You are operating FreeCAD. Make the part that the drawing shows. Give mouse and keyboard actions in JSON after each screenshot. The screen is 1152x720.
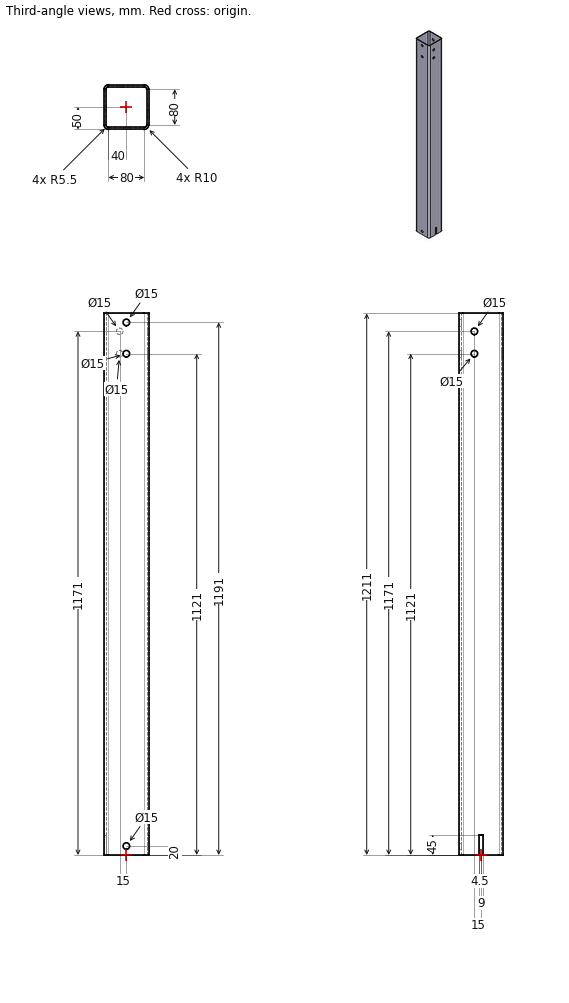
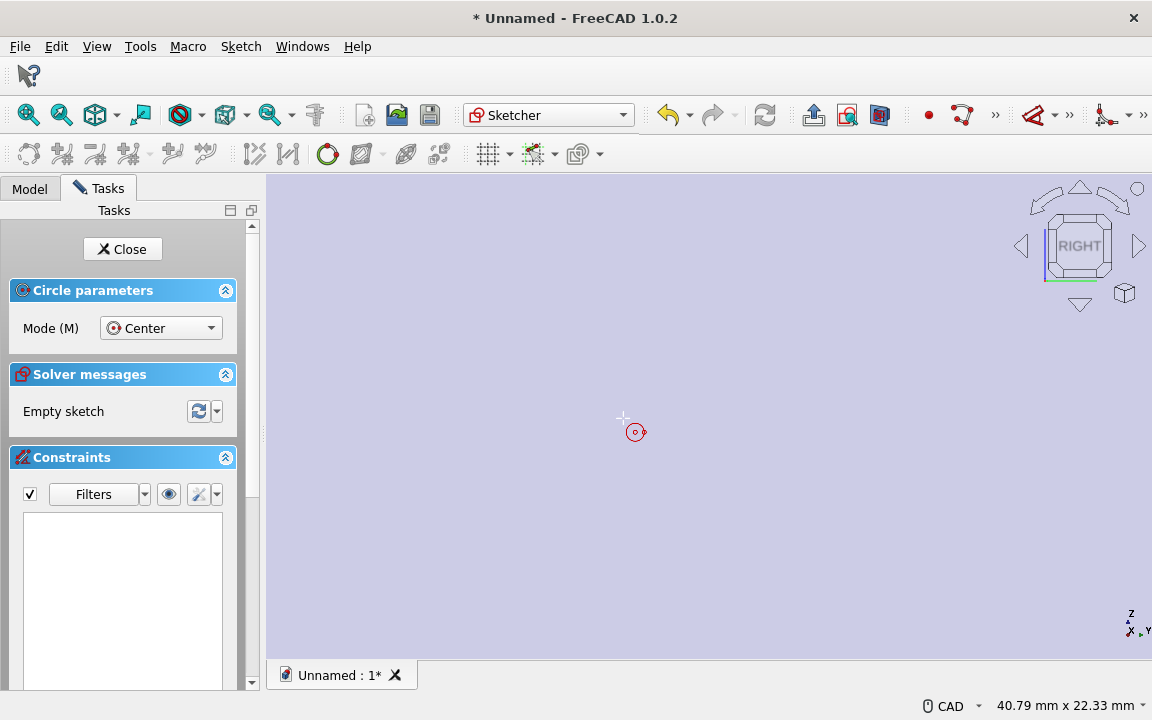
{"action": "left_click", "coordinate": [638, 416]}
{"action": "left_click", "coordinate": [753, 301]}
{"action": "key", "text": "Escape"}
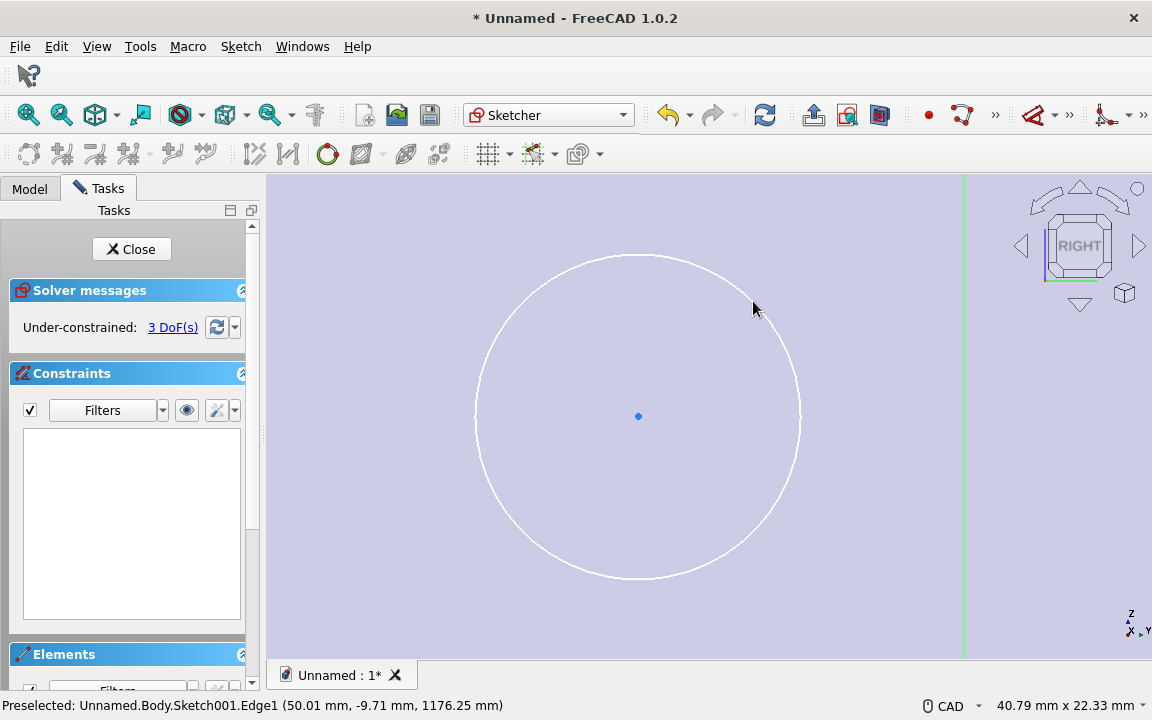
{"action": "key", "text": "d"}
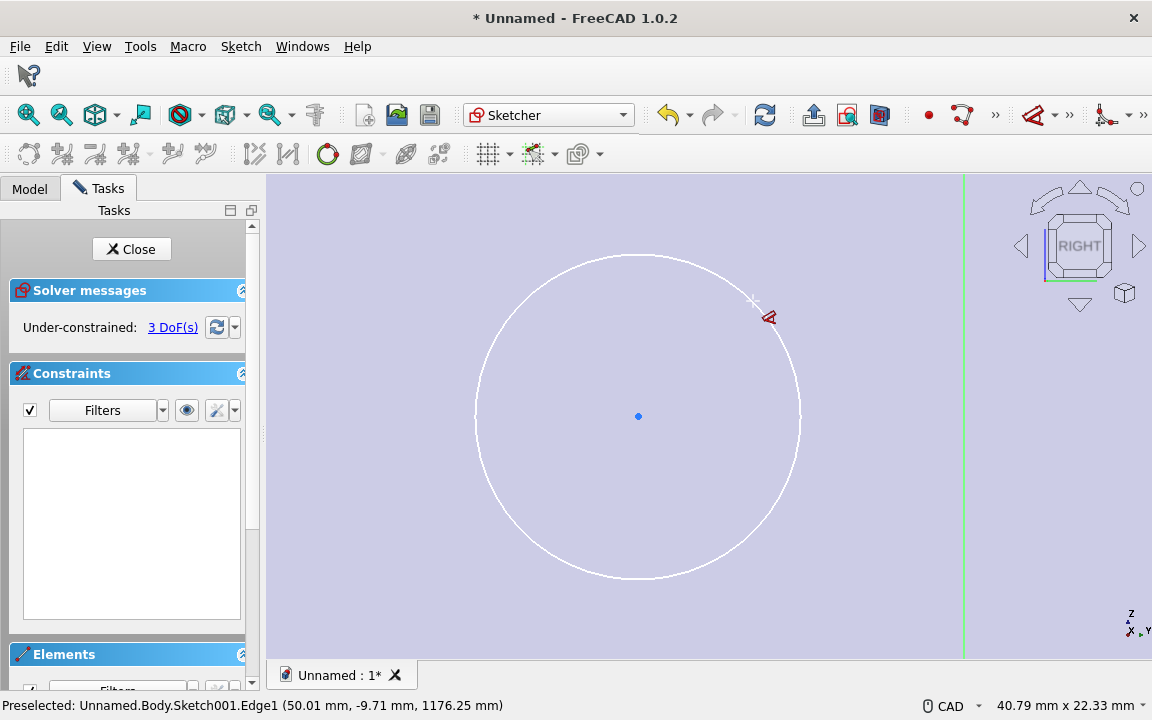
{"action": "left_click", "coordinate": [753, 302]}
{"action": "left_click", "coordinate": [776, 279]}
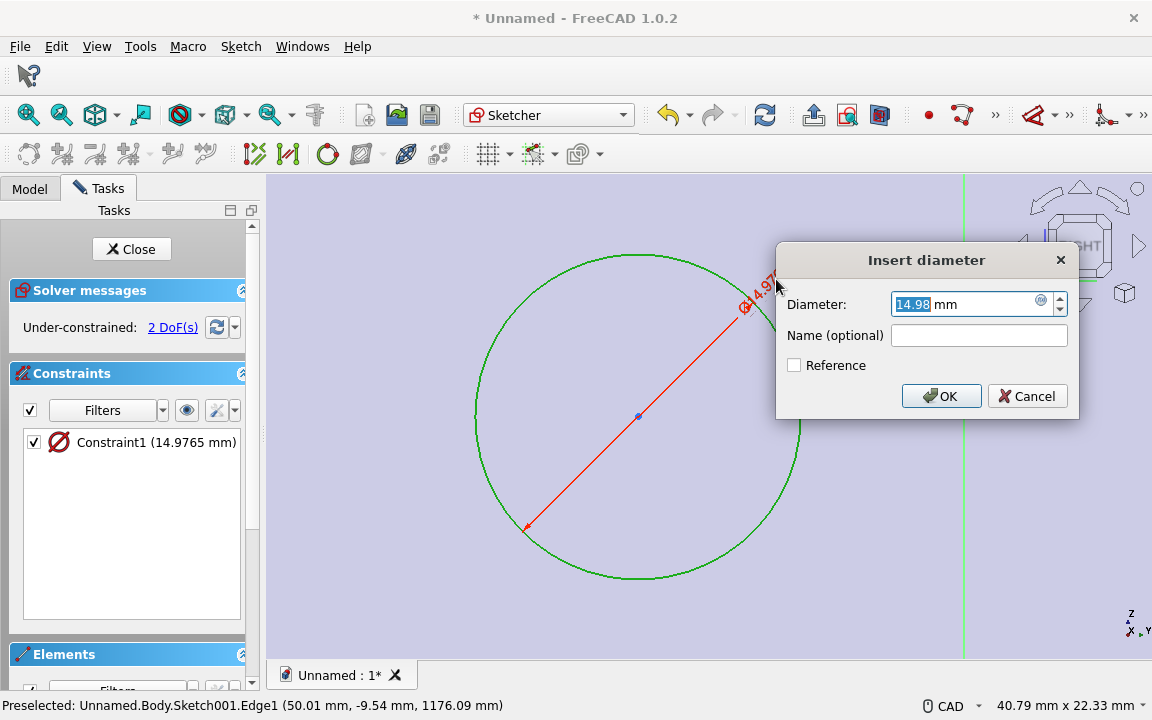
{"action": "type", "text": "15"}
{"action": "key", "text": "Return"}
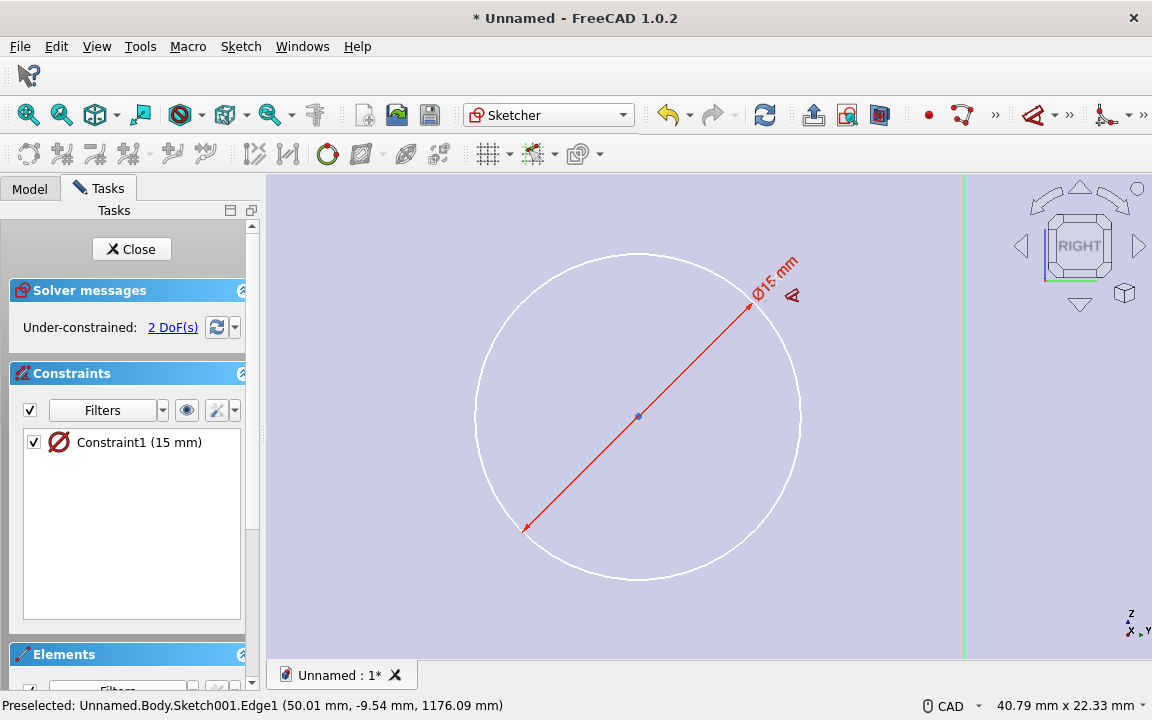
{"action": "left_click", "coordinate": [638, 417]}
{"action": "left_click", "coordinate": [726, 383]}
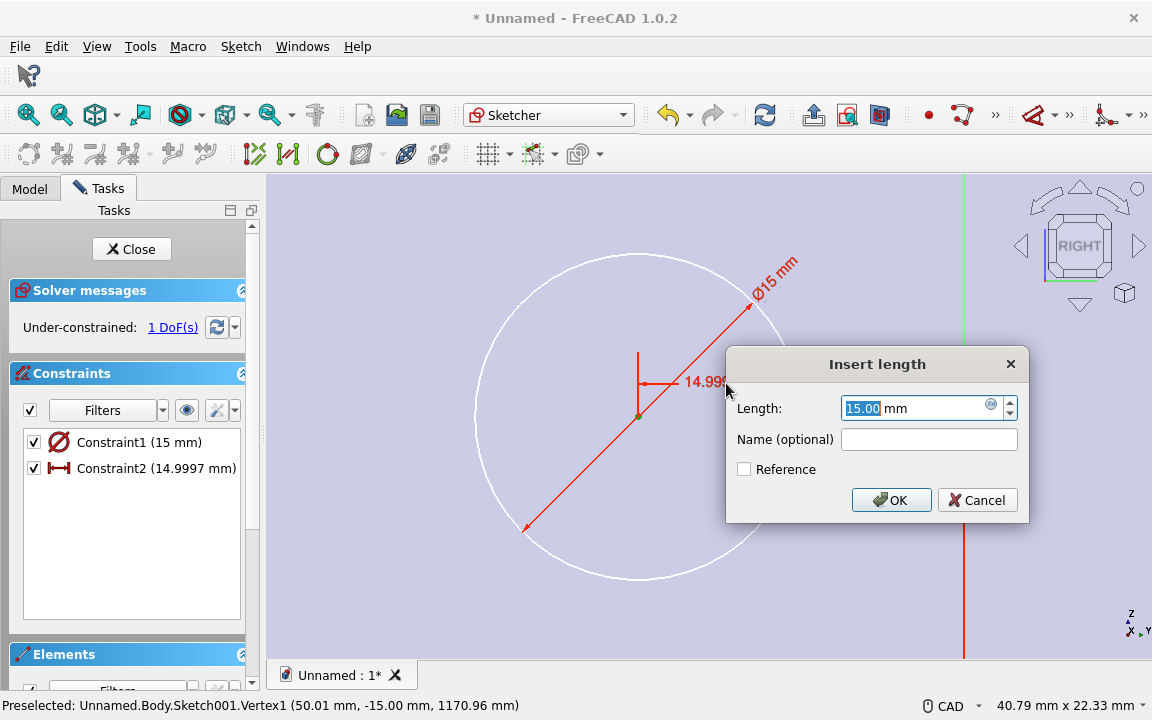
{"action": "type", "text": "15"}
{"action": "key", "text": "Return"}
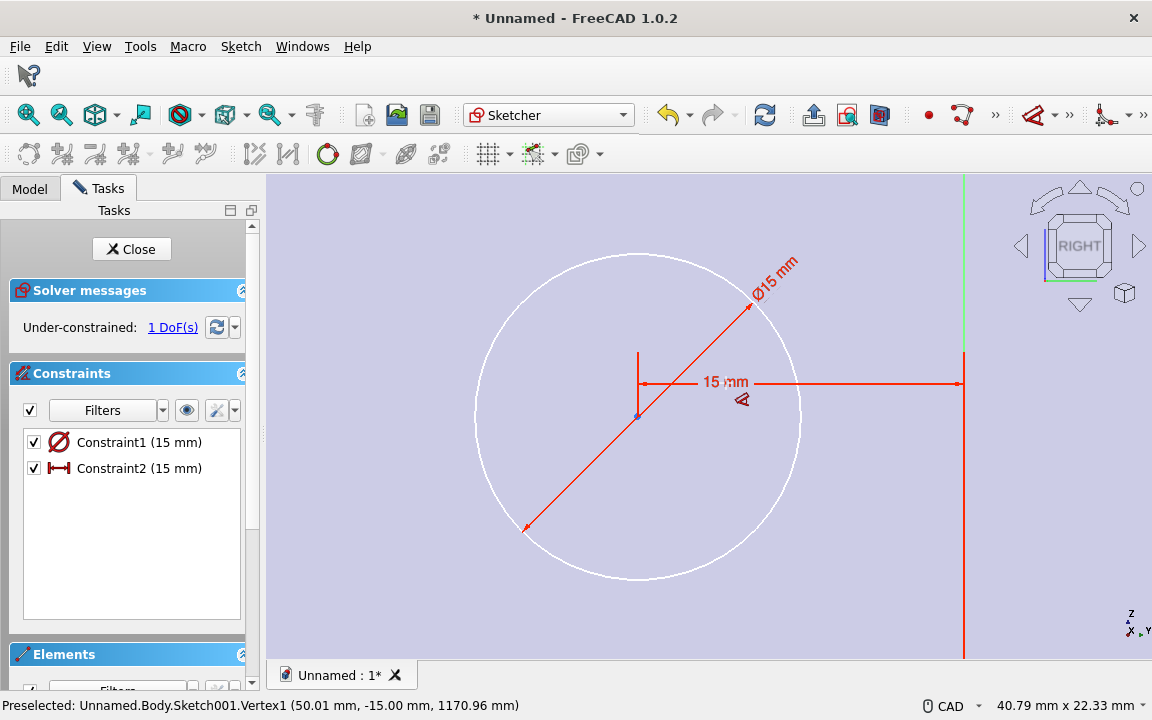
{"action": "left_click", "coordinate": [638, 417]}
{"action": "left_click", "coordinate": [604, 524]}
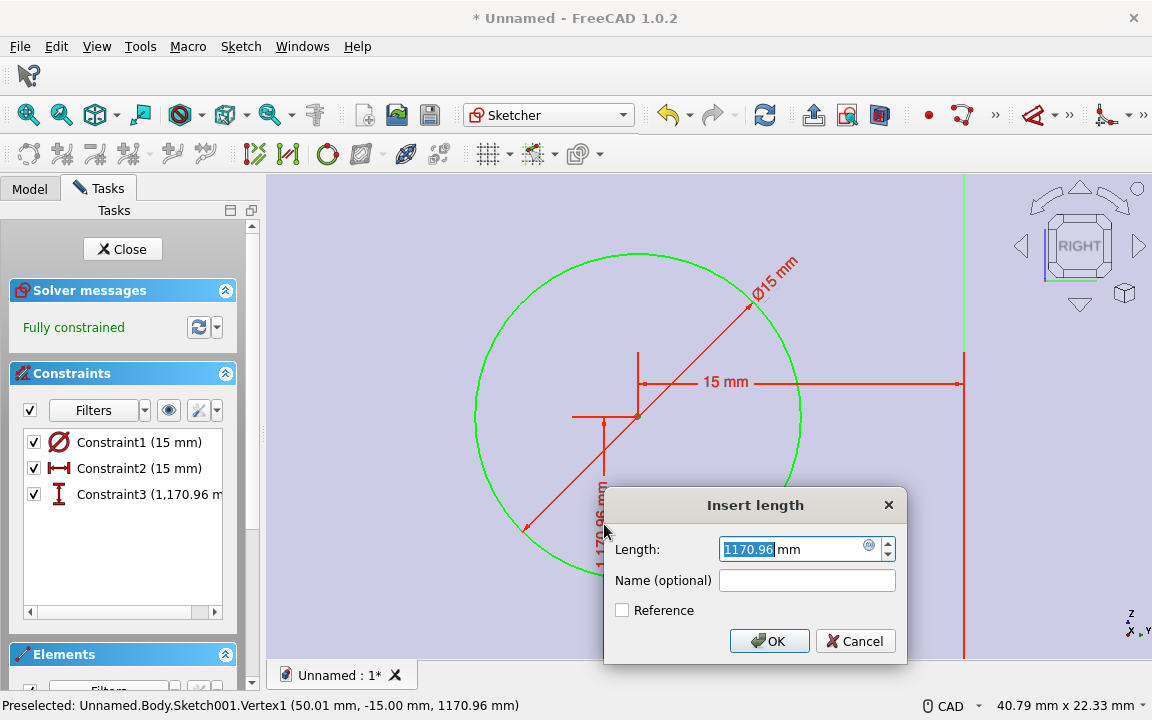
{"action": "type", "text": "1171"}
{"action": "key", "text": "Return"}
{"action": "key", "text": "Escape"}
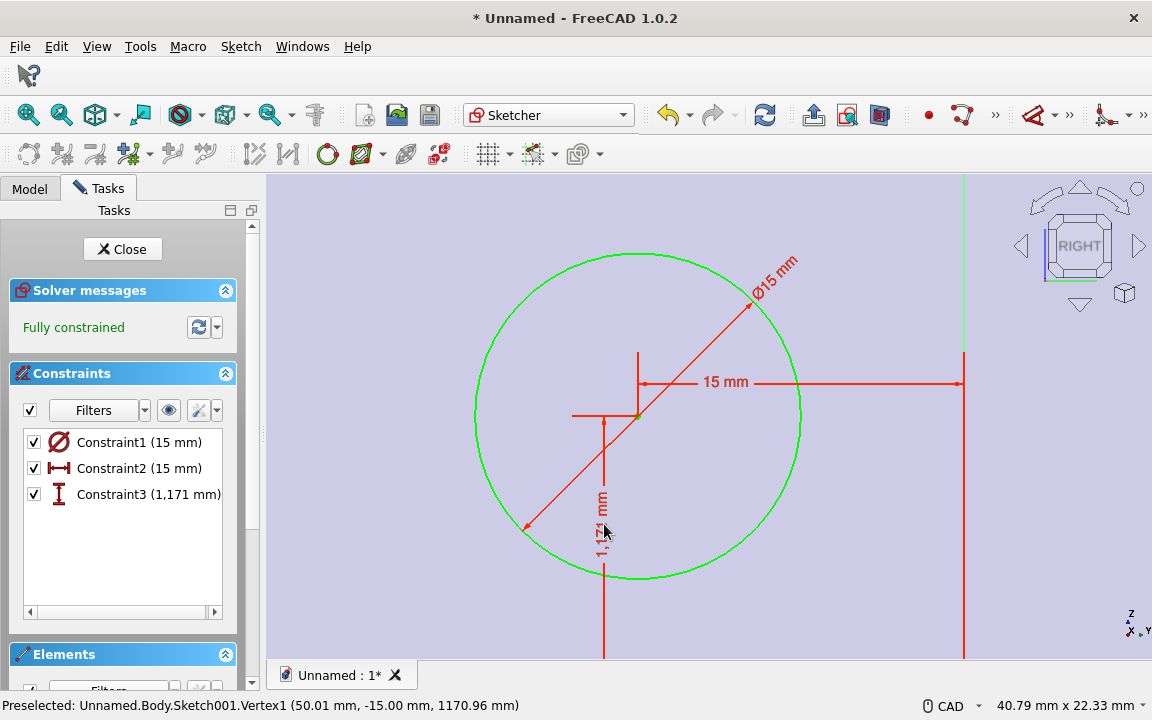
{"action": "left_click", "coordinate": [123, 249]}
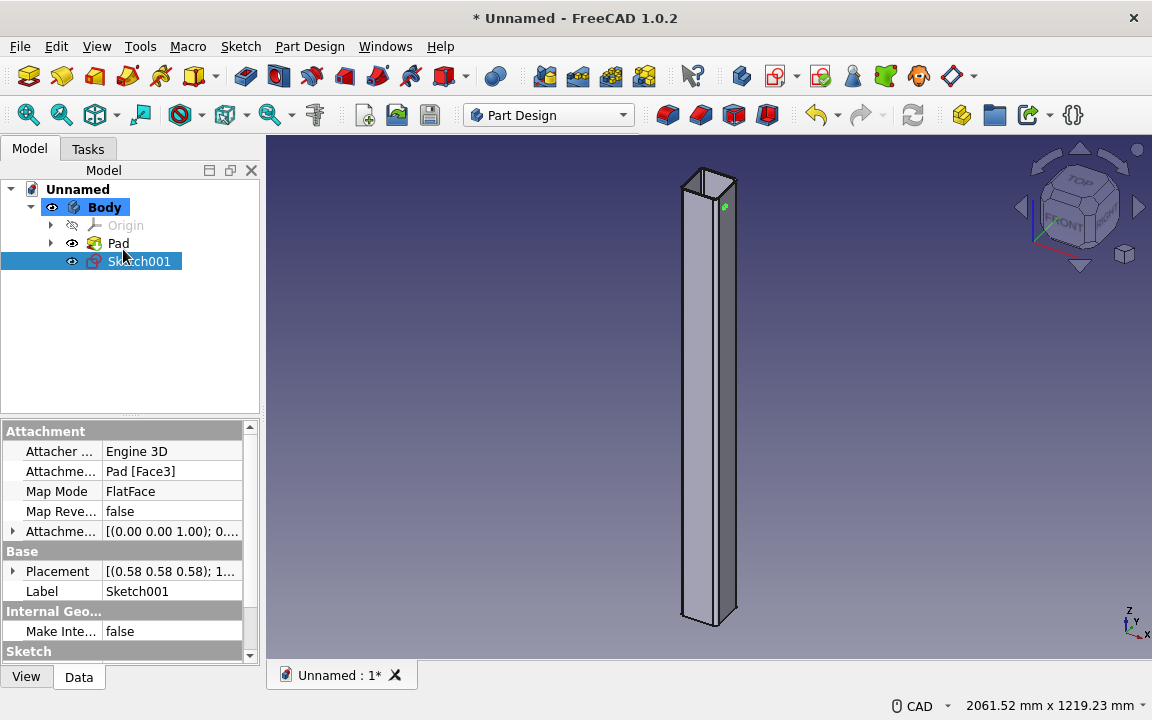
{"action": "left_click", "coordinate": [246, 76]}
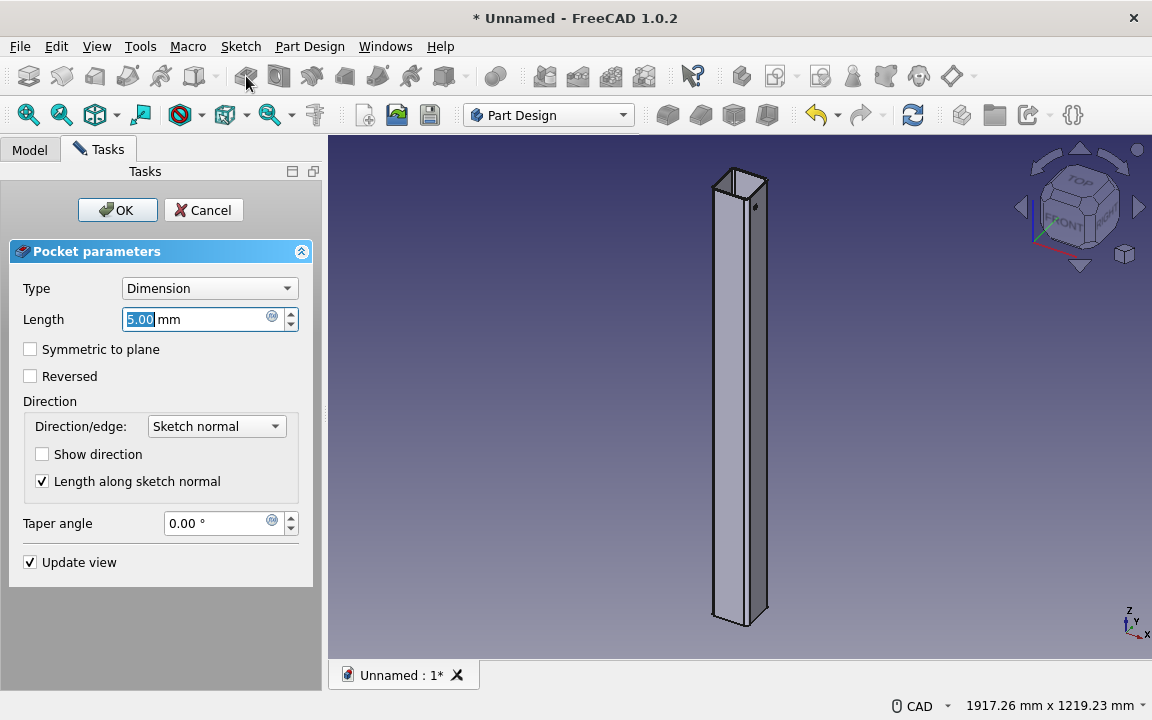
{"action": "left_click", "coordinate": [210, 288]}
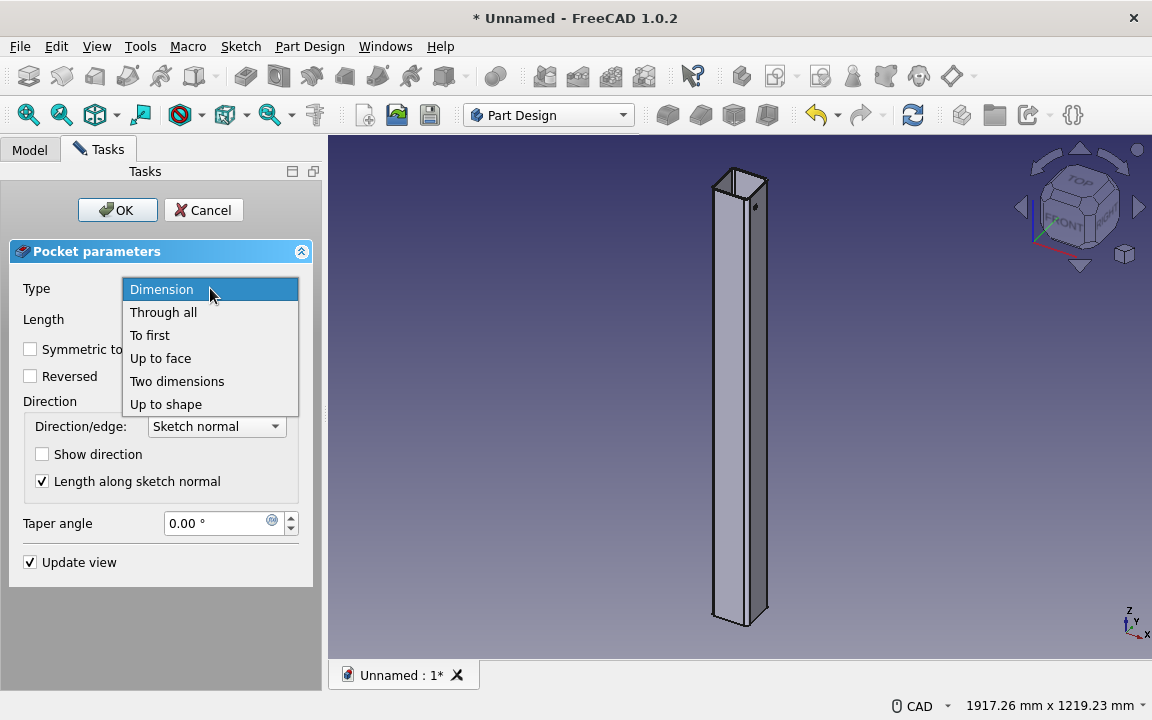
{"action": "left_click", "coordinate": [208, 336]}